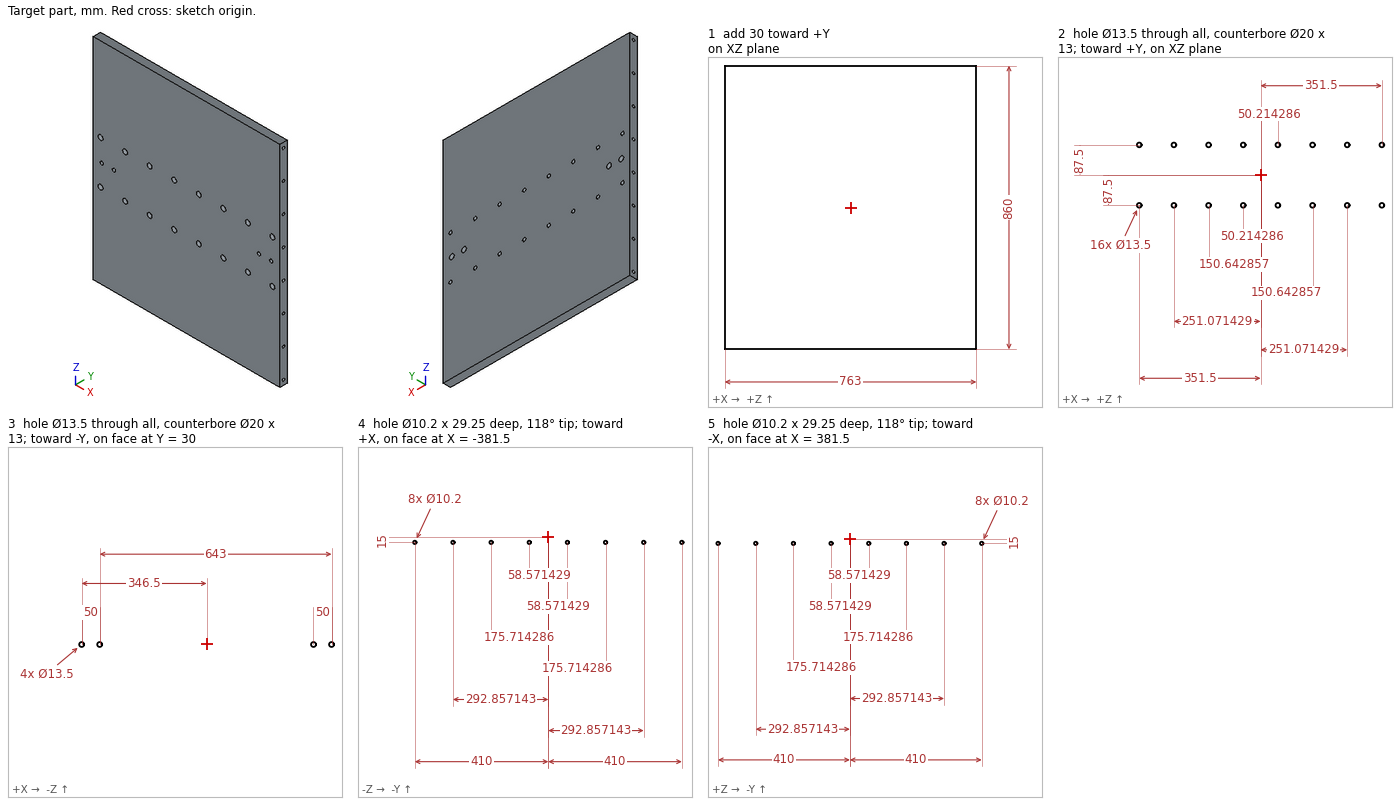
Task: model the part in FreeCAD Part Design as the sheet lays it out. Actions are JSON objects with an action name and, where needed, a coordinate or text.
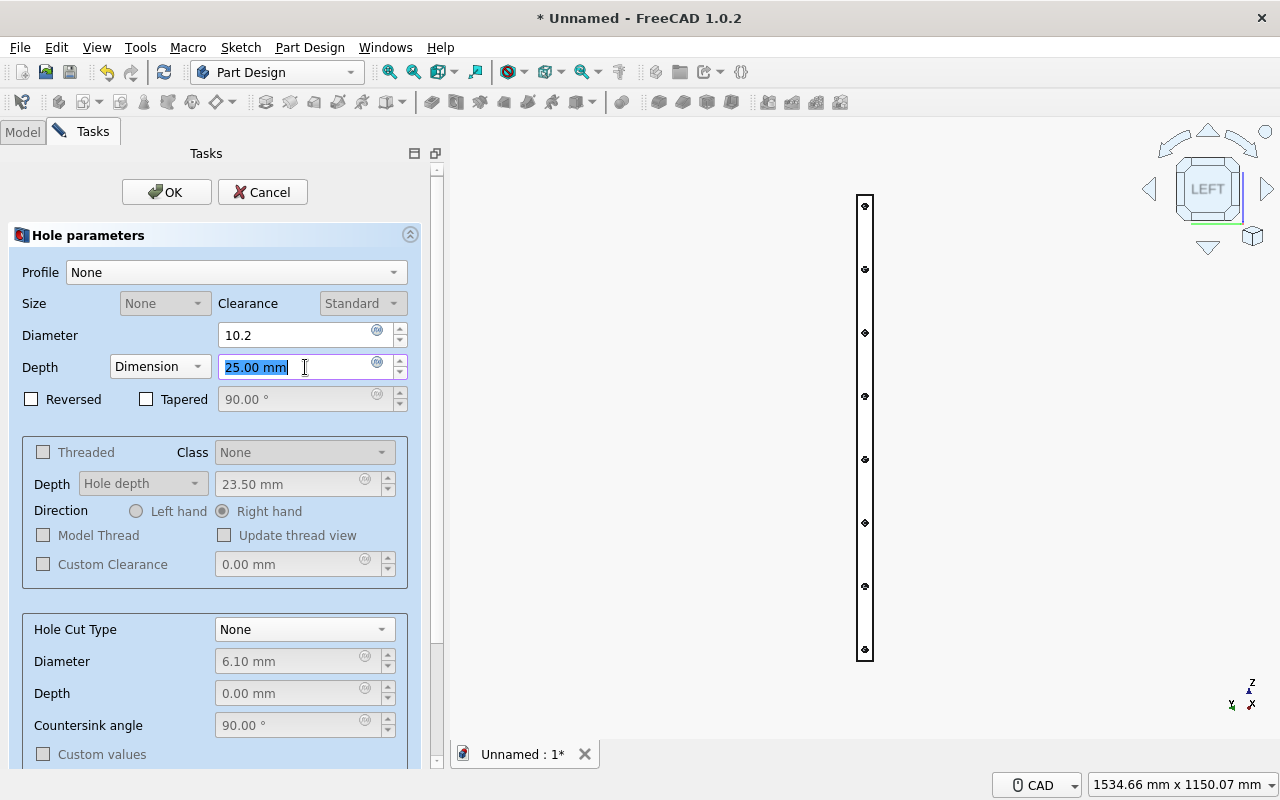
{"action": "type", "text": "29.25"}
{"action": "key", "text": "Tab"}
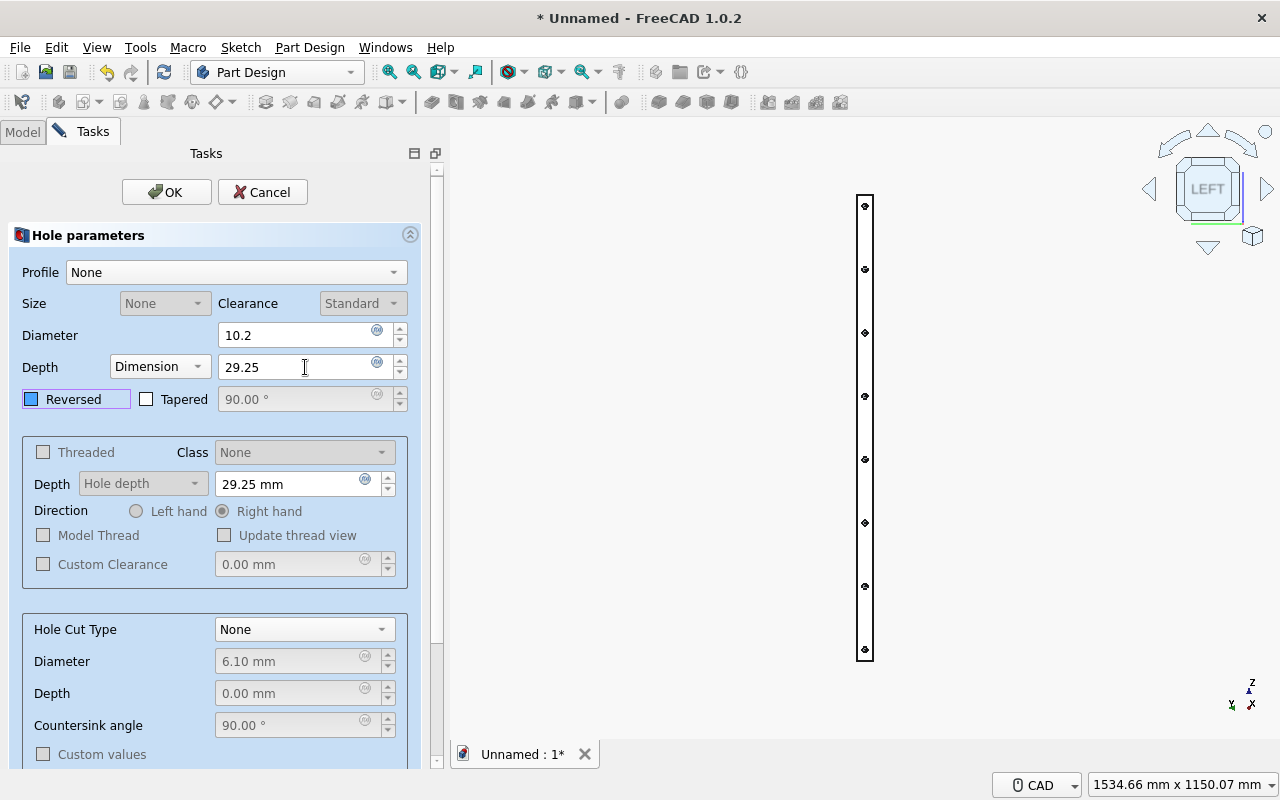
{"action": "left_click", "coordinate": [167, 192]}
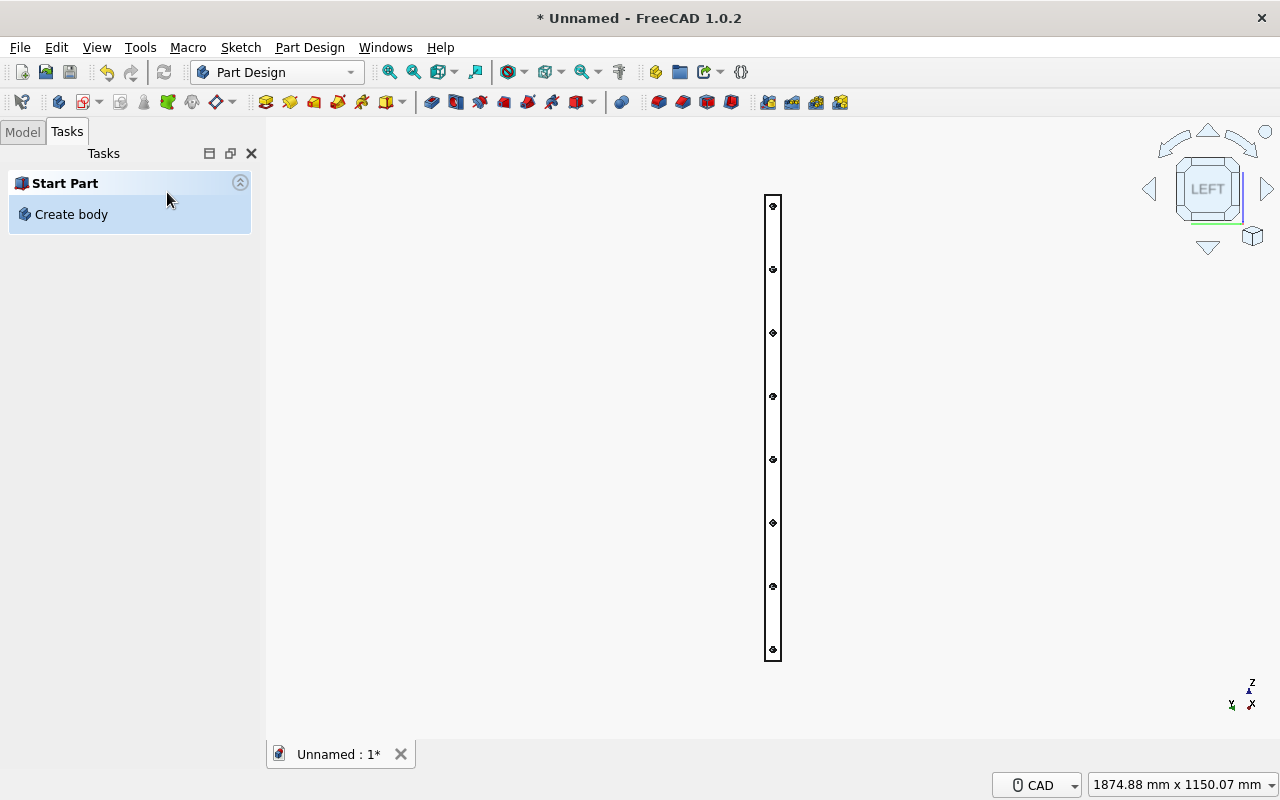
{"action": "key", "text": "0"}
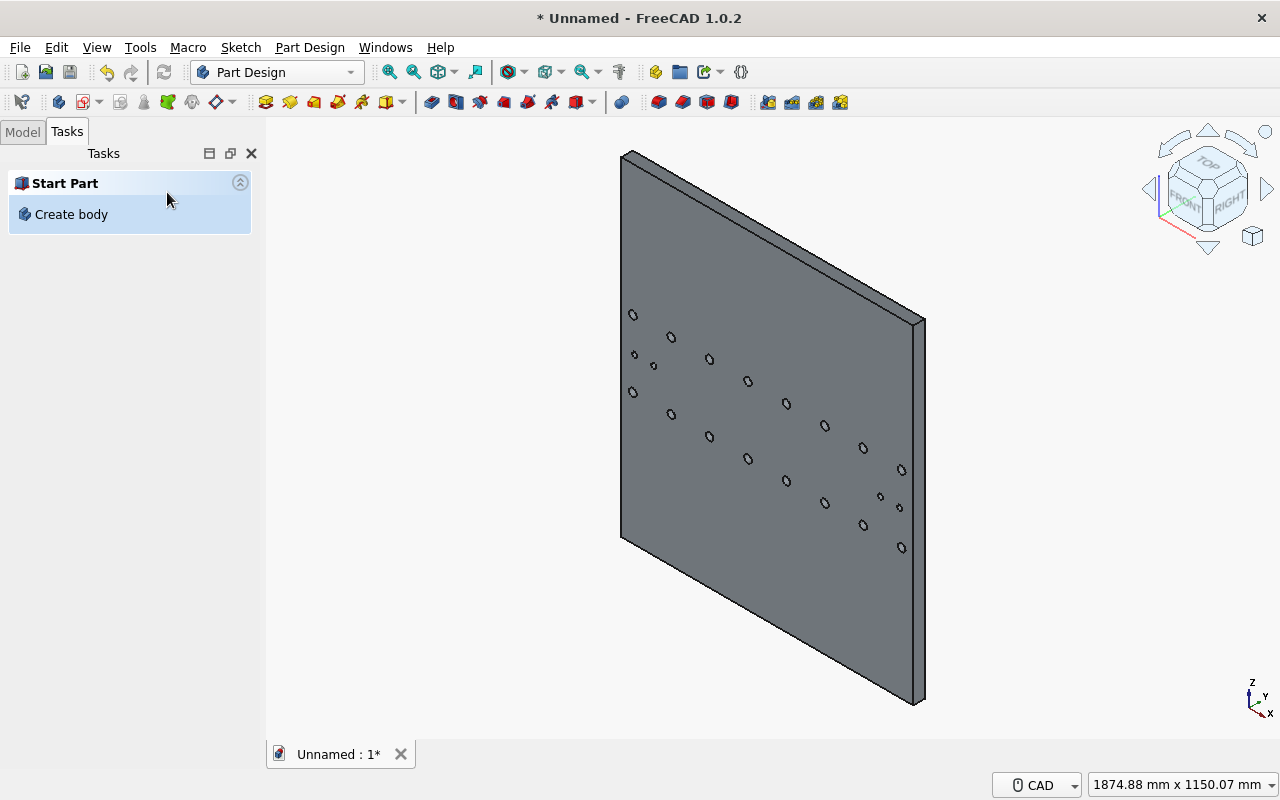
{"action": "key", "text": "3"}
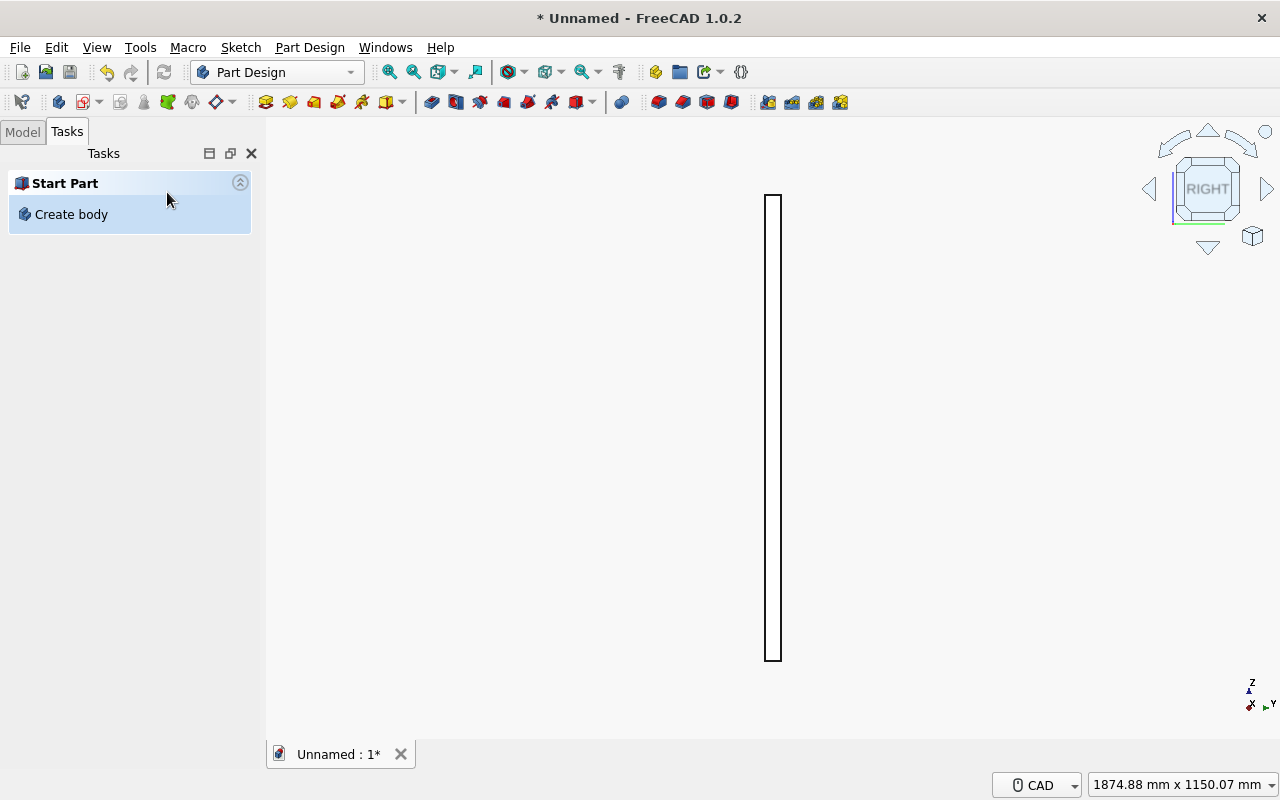
{"action": "left_click", "coordinate": [773, 228]}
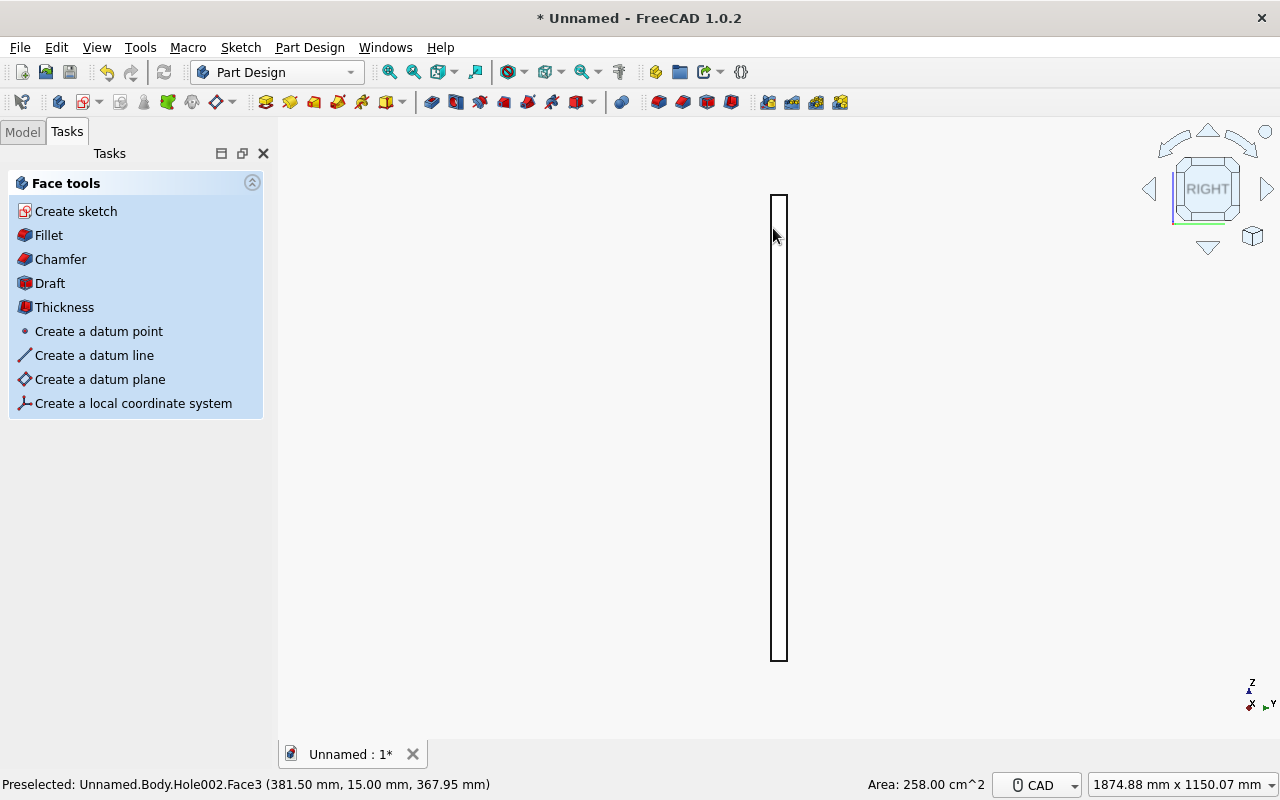
{"action": "left_click", "coordinate": [84, 102]}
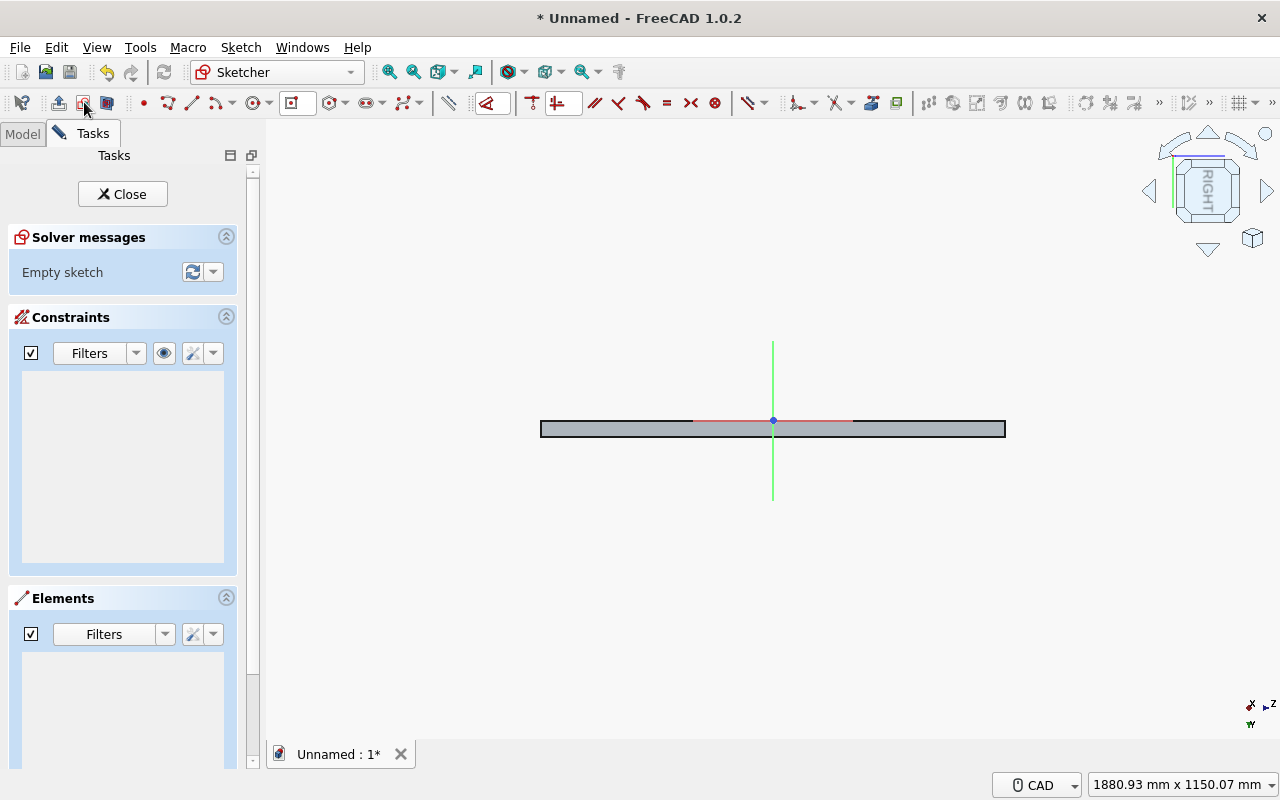
{"action": "left_click", "coordinate": [254, 104]}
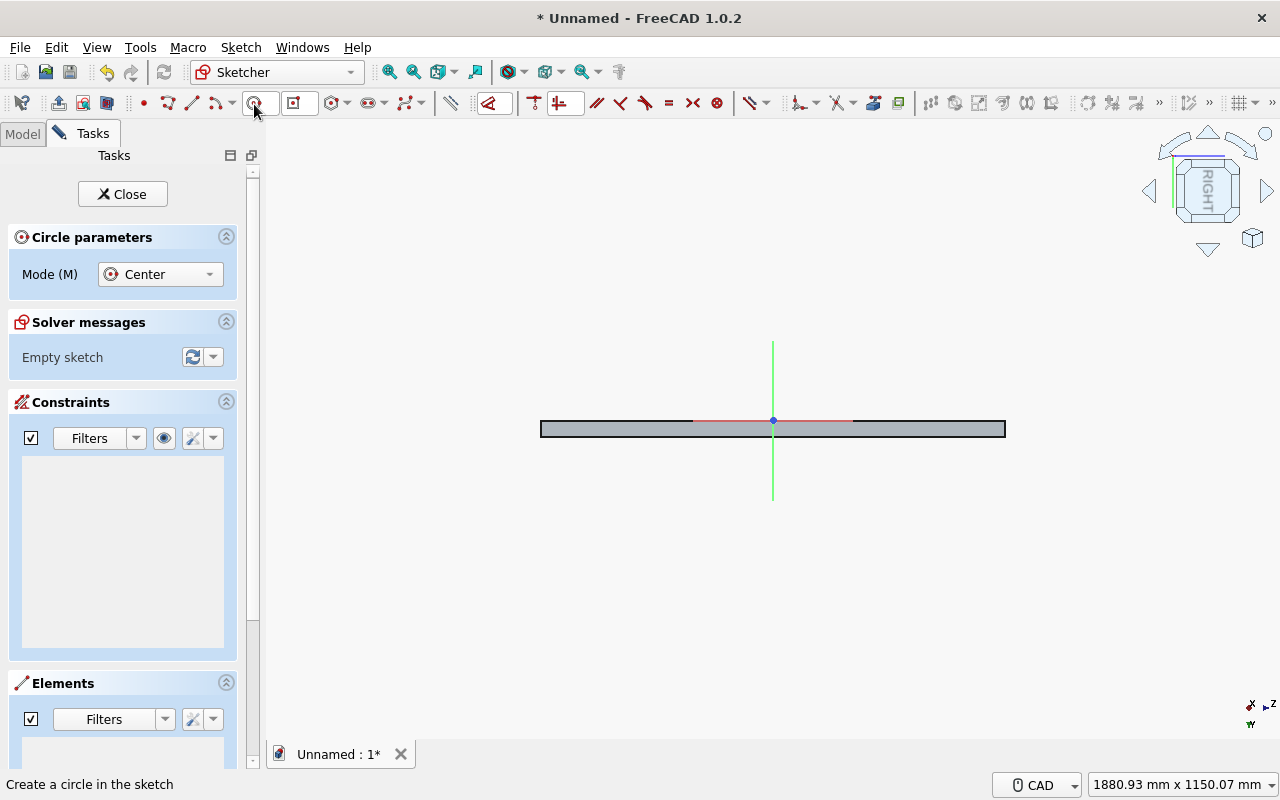
{"action": "scroll", "coordinate": [994, 429], "scroll_direction": "up", "scroll_amount": 11}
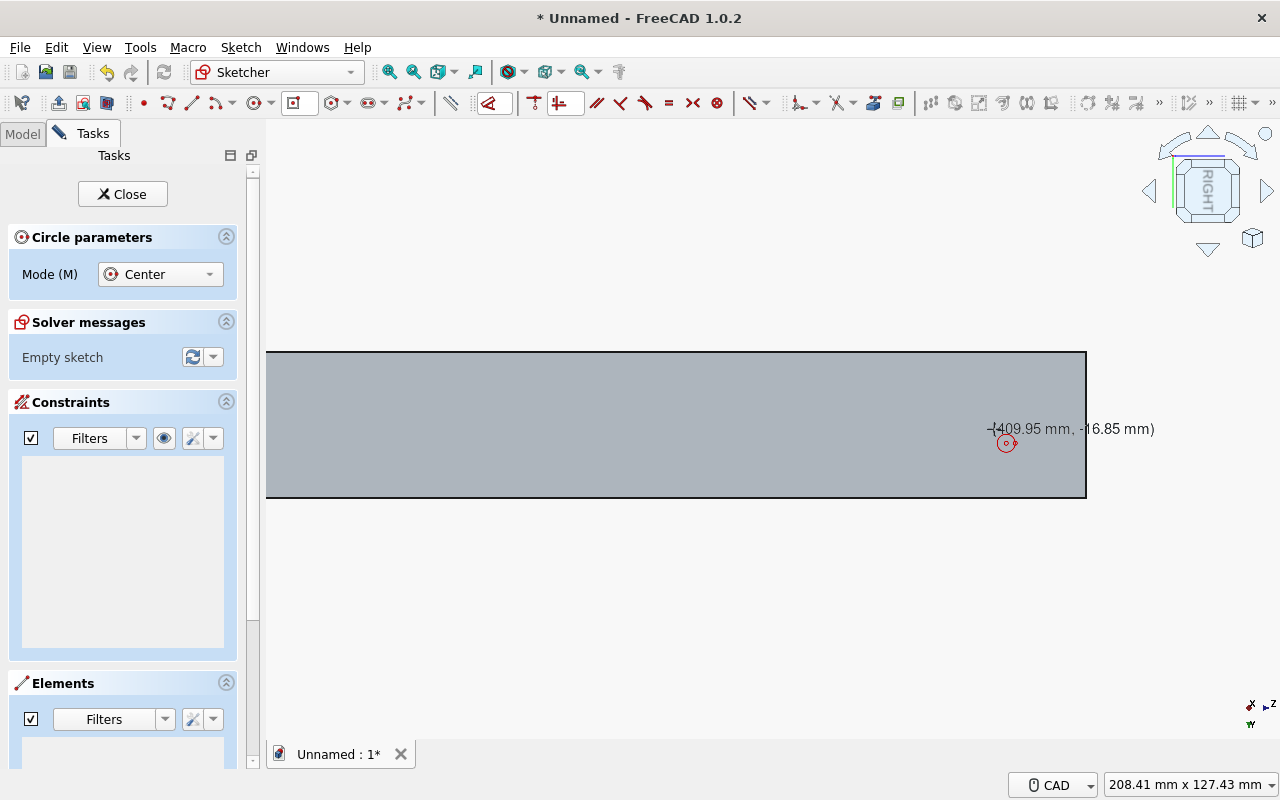
{"action": "scroll", "coordinate": [972, 433], "scroll_direction": "down", "scroll_amount": 10}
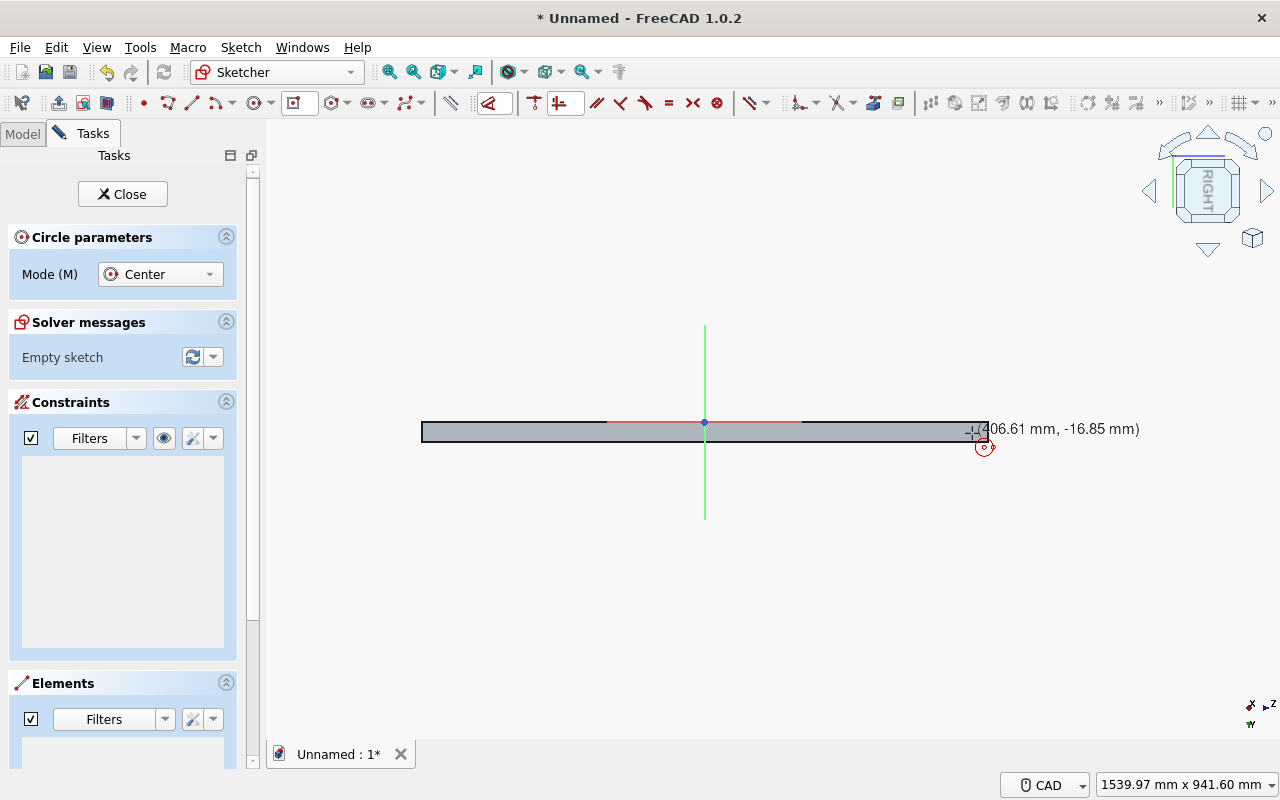
{"action": "scroll", "coordinate": [975, 432], "scroll_direction": "up", "scroll_amount": 3}